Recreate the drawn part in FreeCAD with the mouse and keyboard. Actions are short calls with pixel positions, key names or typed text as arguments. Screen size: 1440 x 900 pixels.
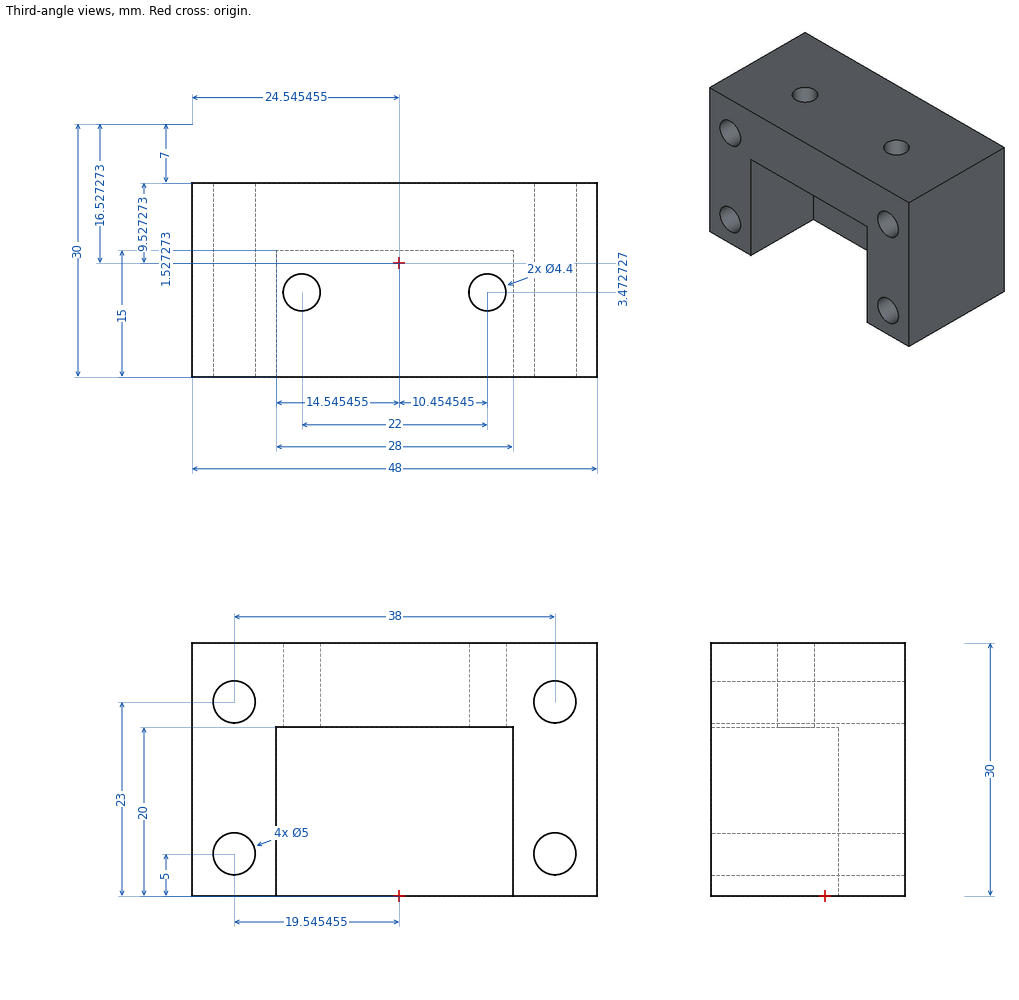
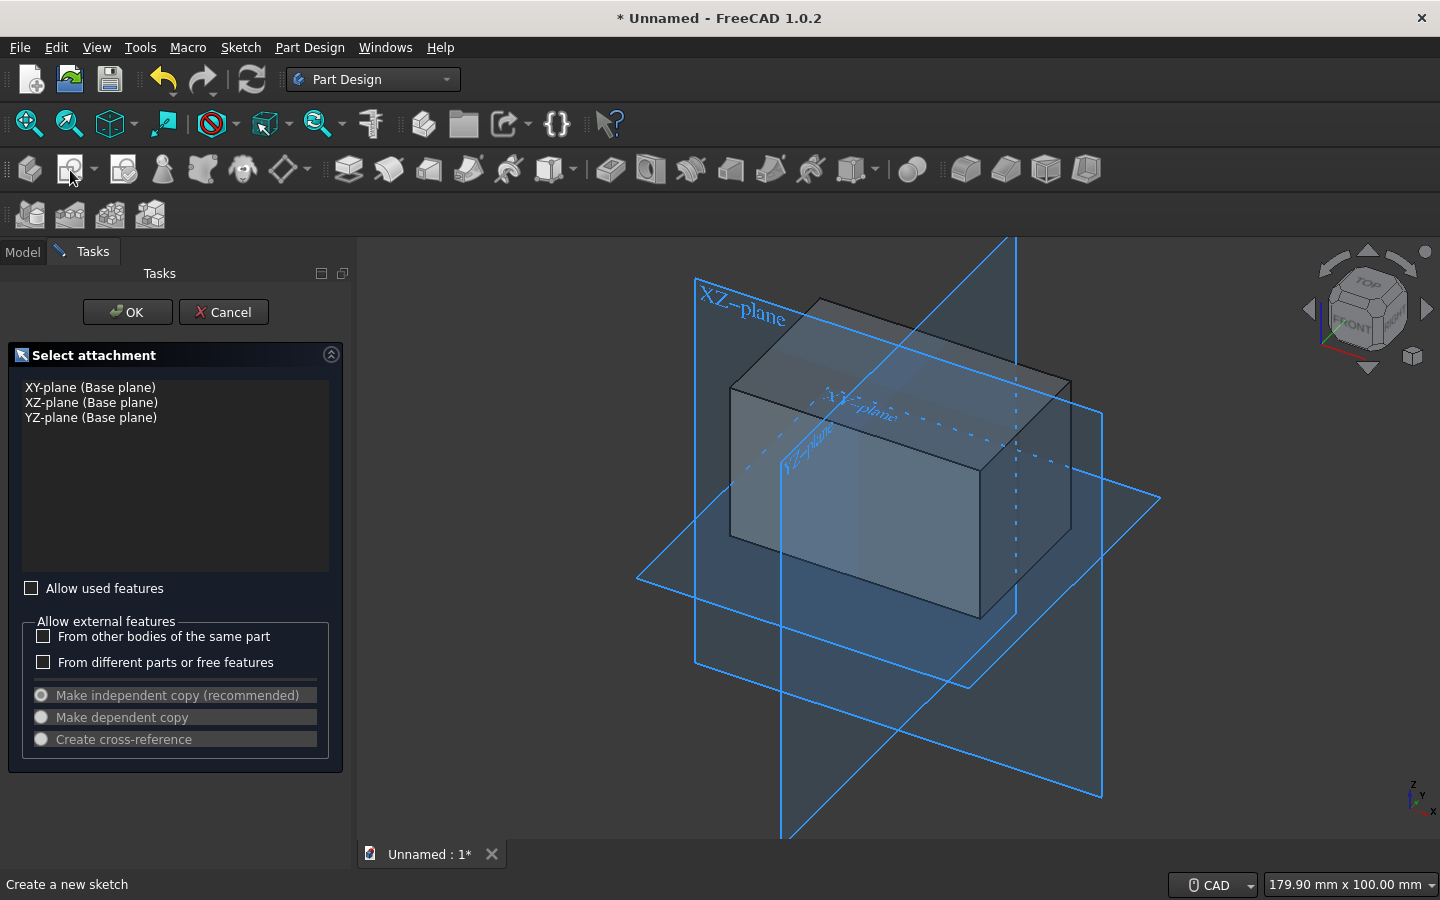
click(82, 388)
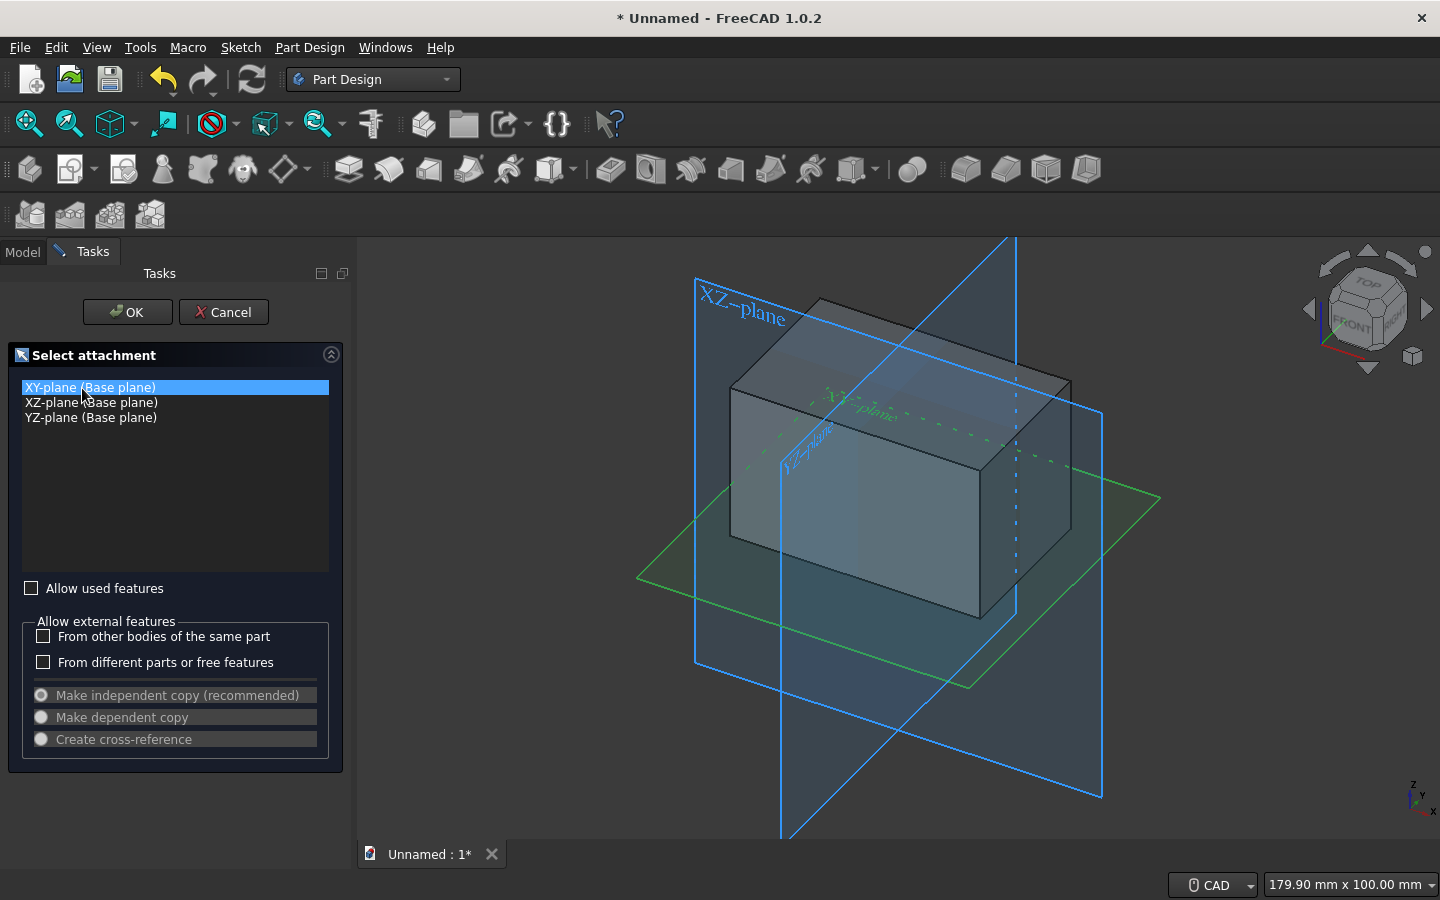
click(128, 312)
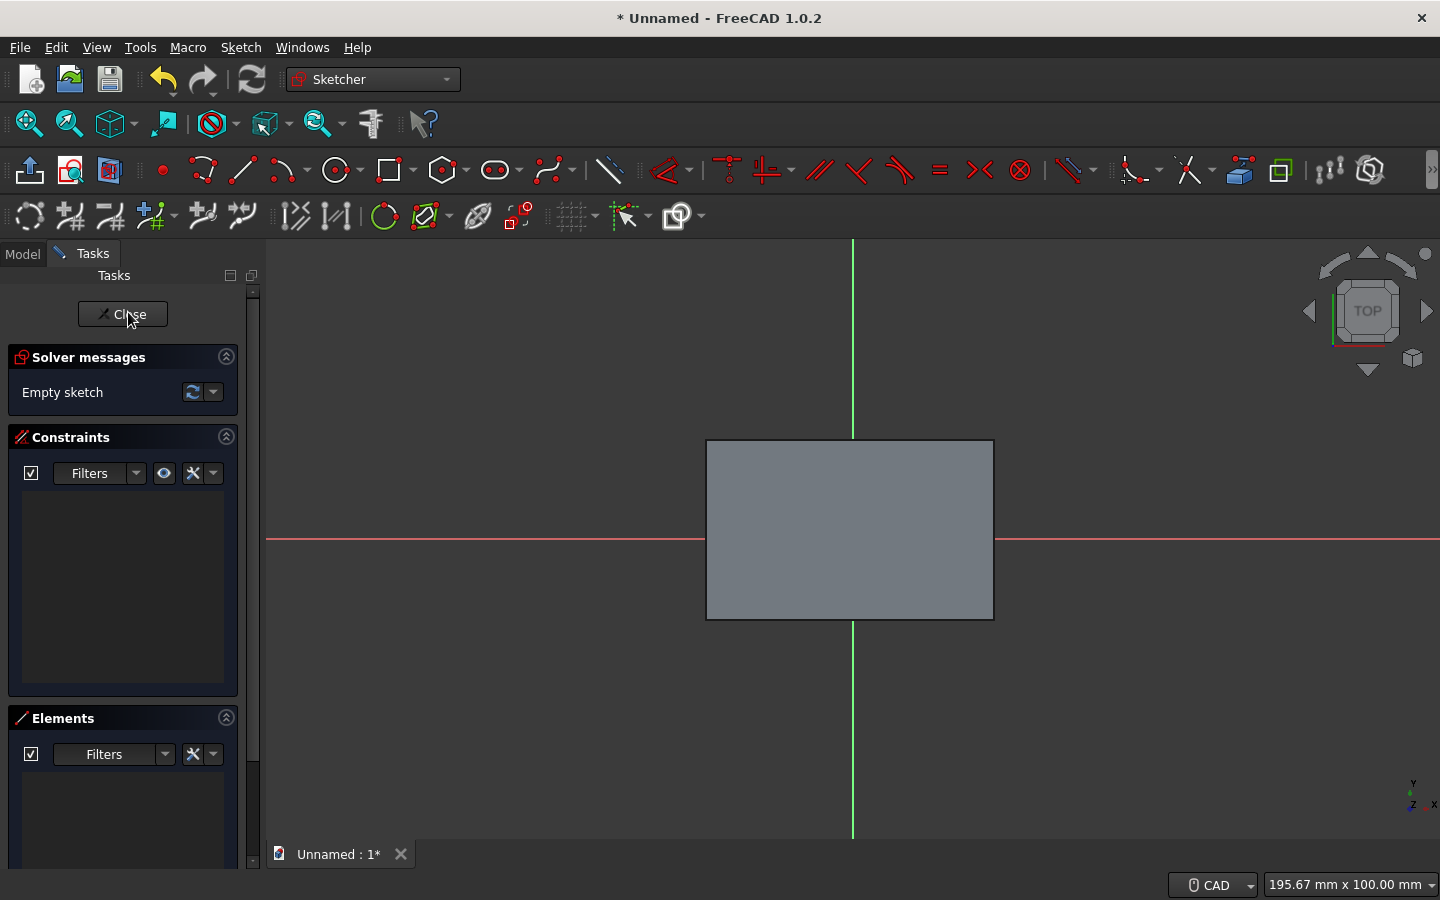
click(110, 170)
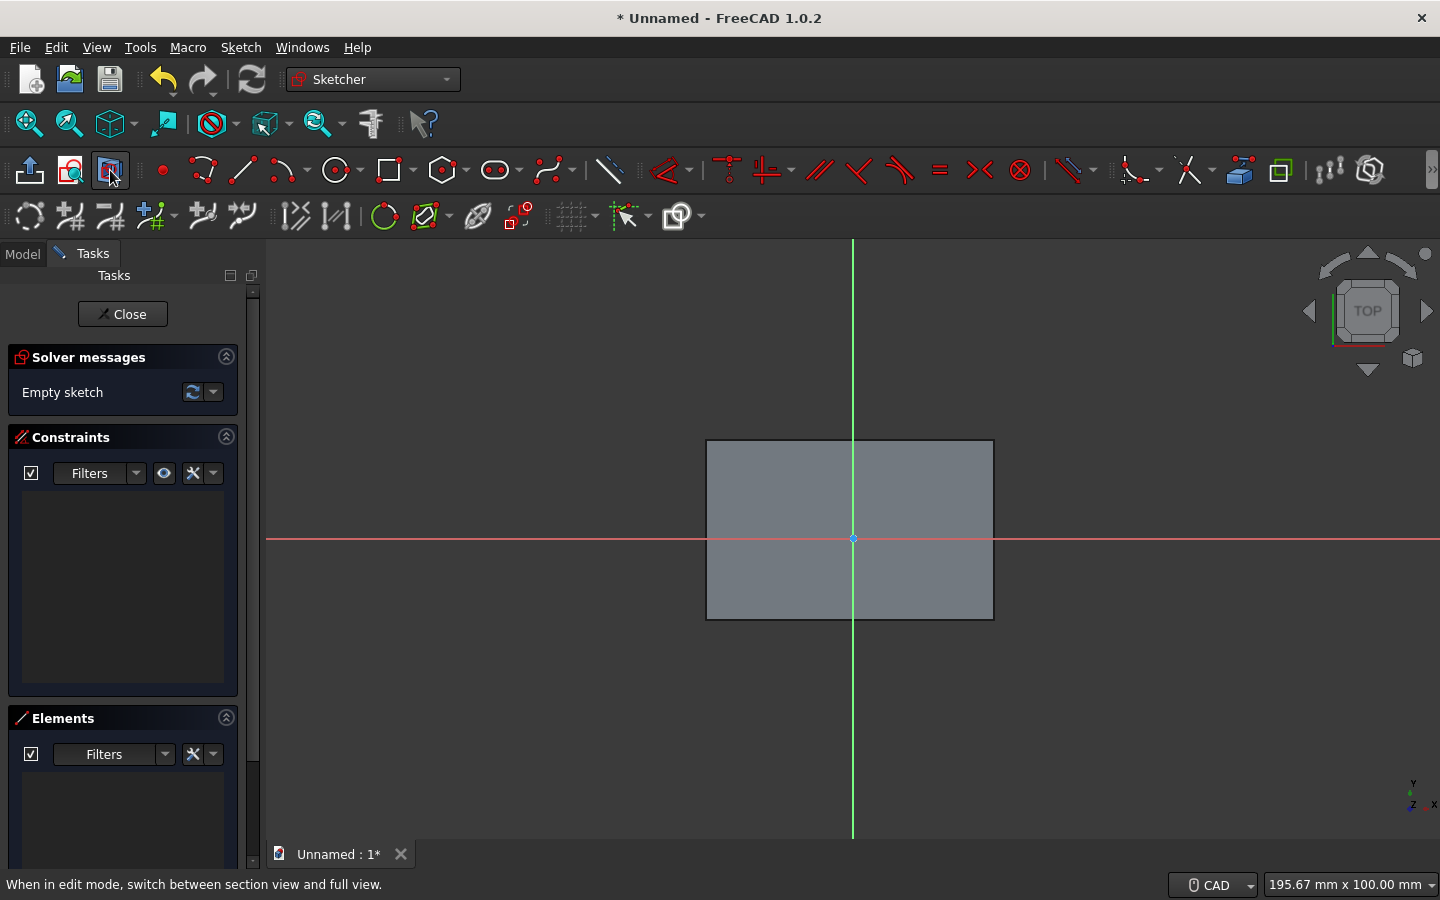
scroll(871, 587, up, 7)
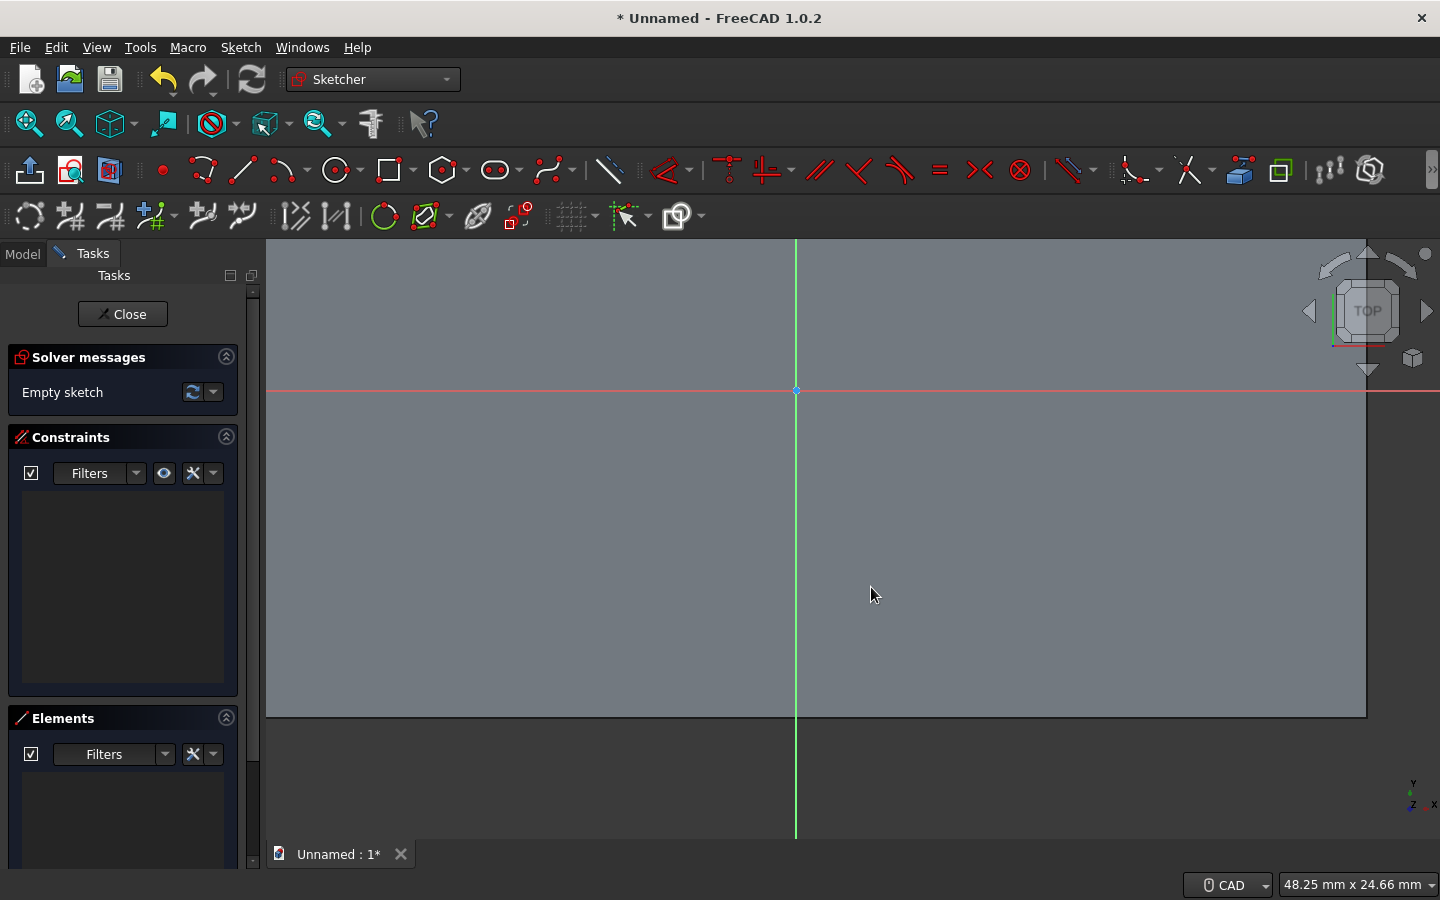
click(390, 170)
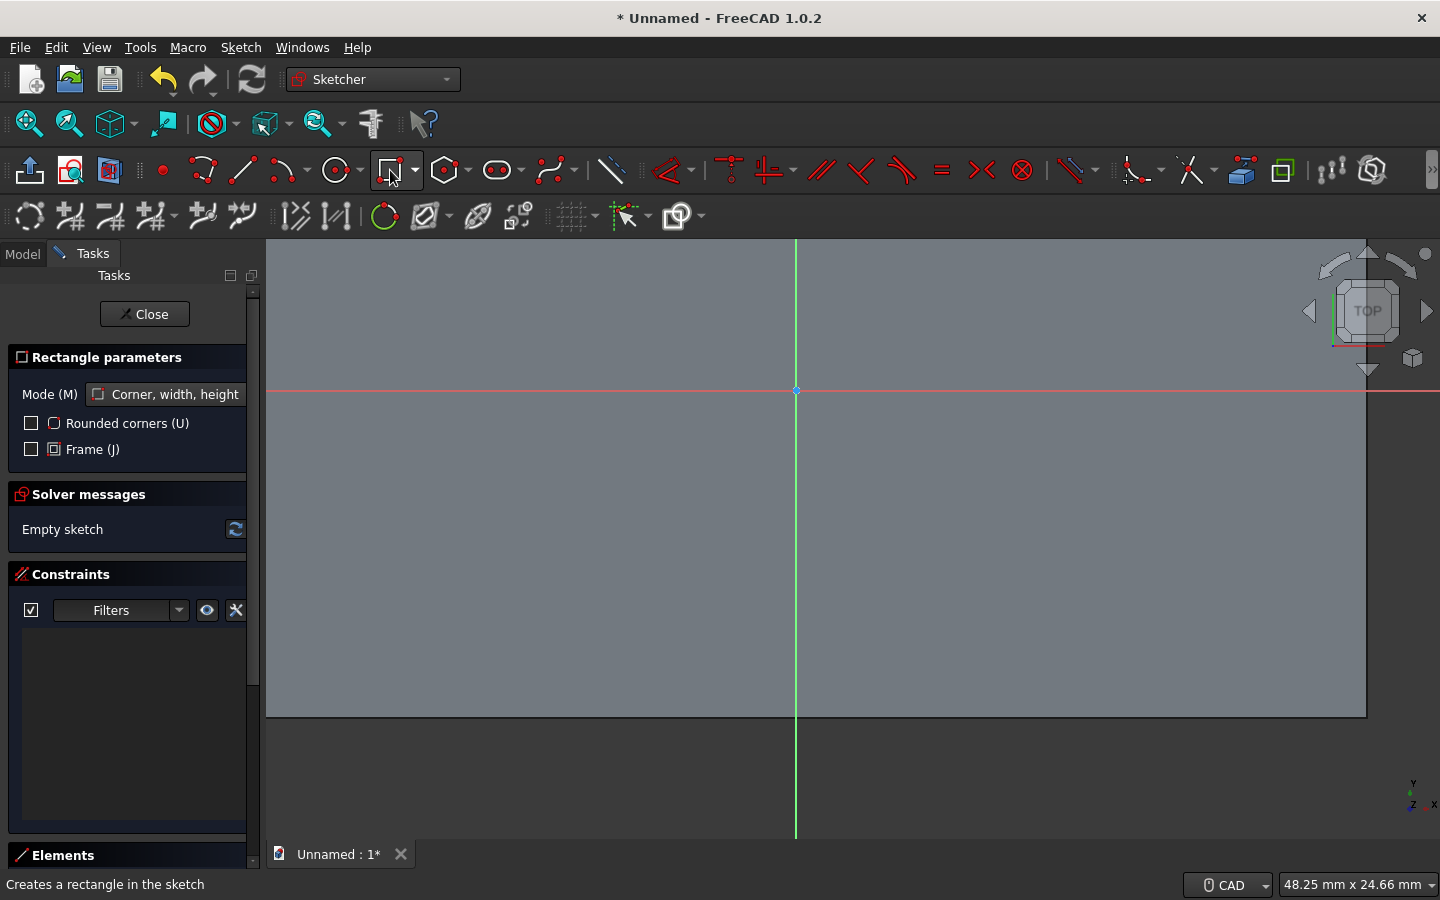
click(443, 353)
click(1124, 718)
key(Escape)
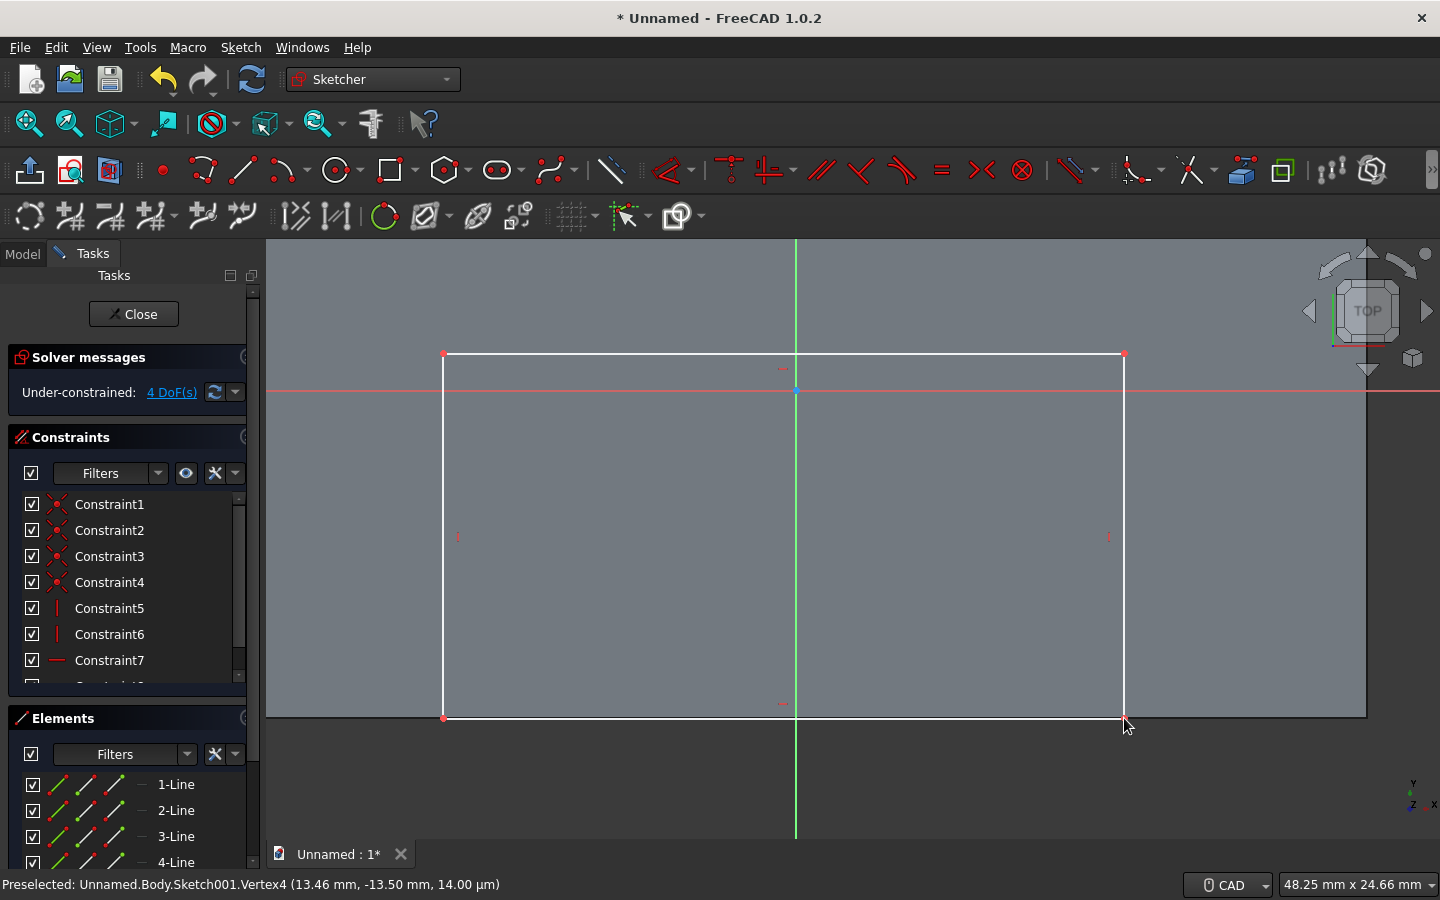
click(666, 170)